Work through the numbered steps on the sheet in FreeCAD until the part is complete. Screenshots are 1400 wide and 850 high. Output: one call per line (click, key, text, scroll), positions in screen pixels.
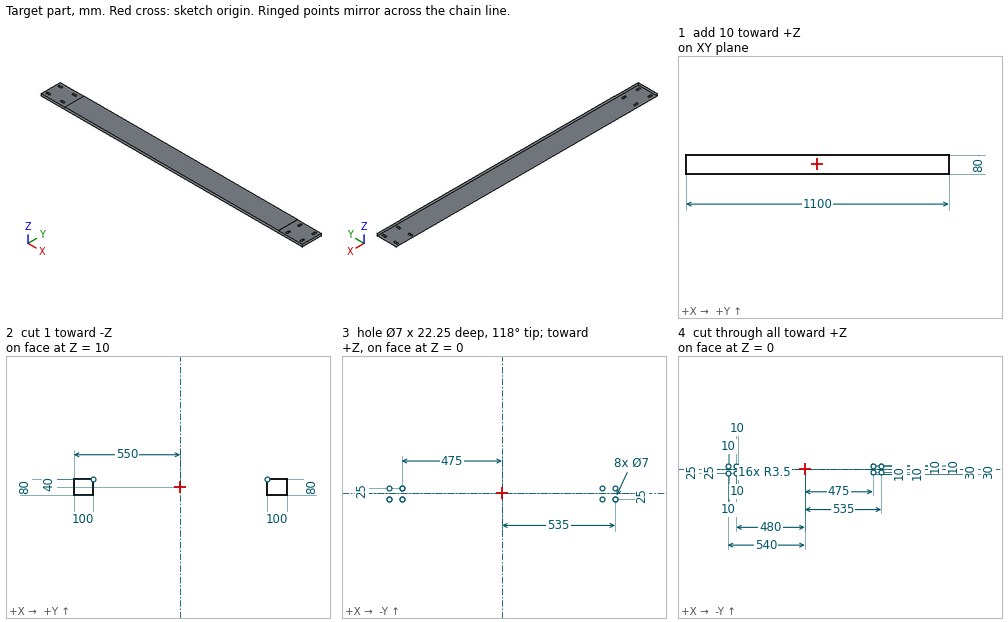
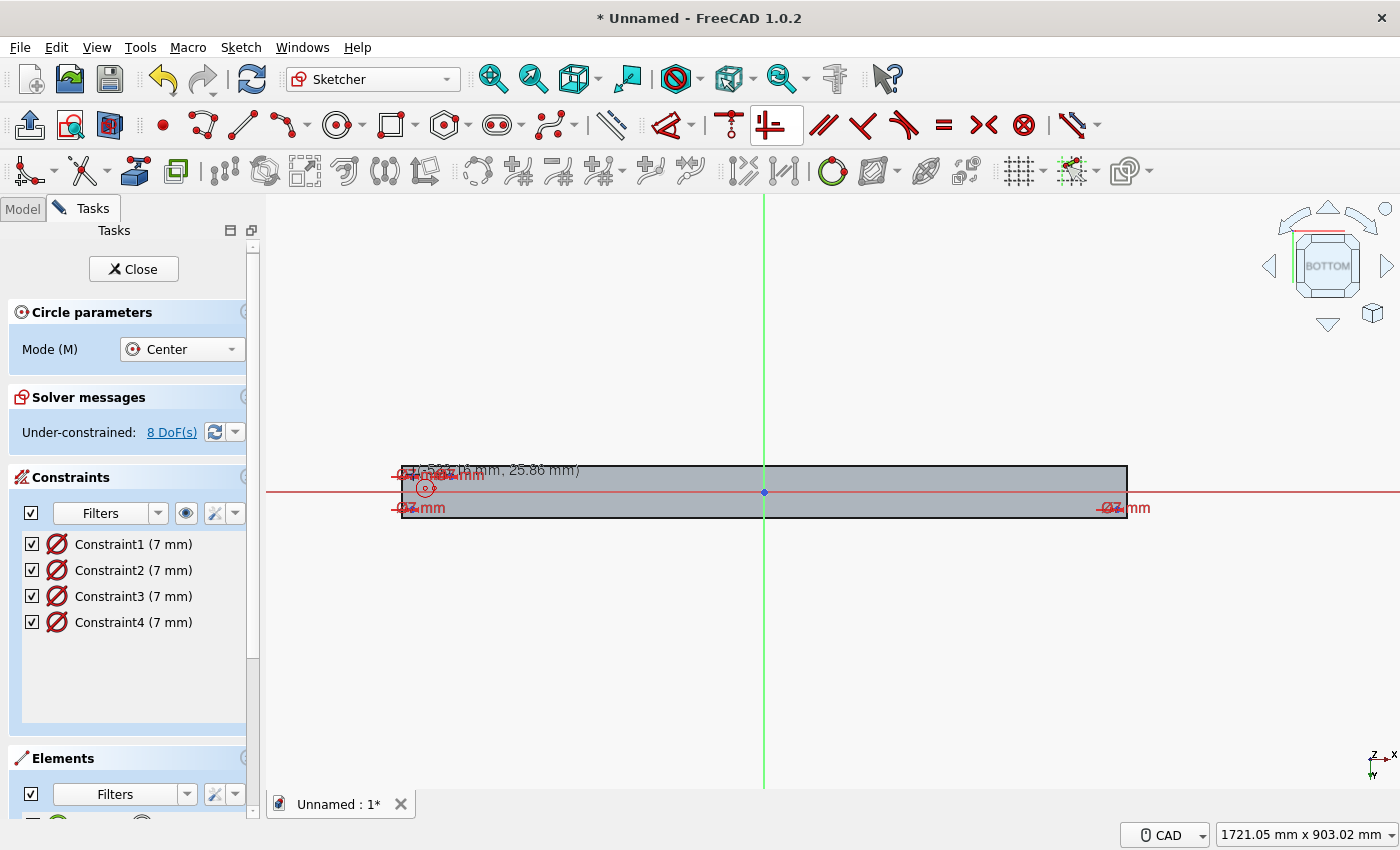
scroll(451, 509, up, 12)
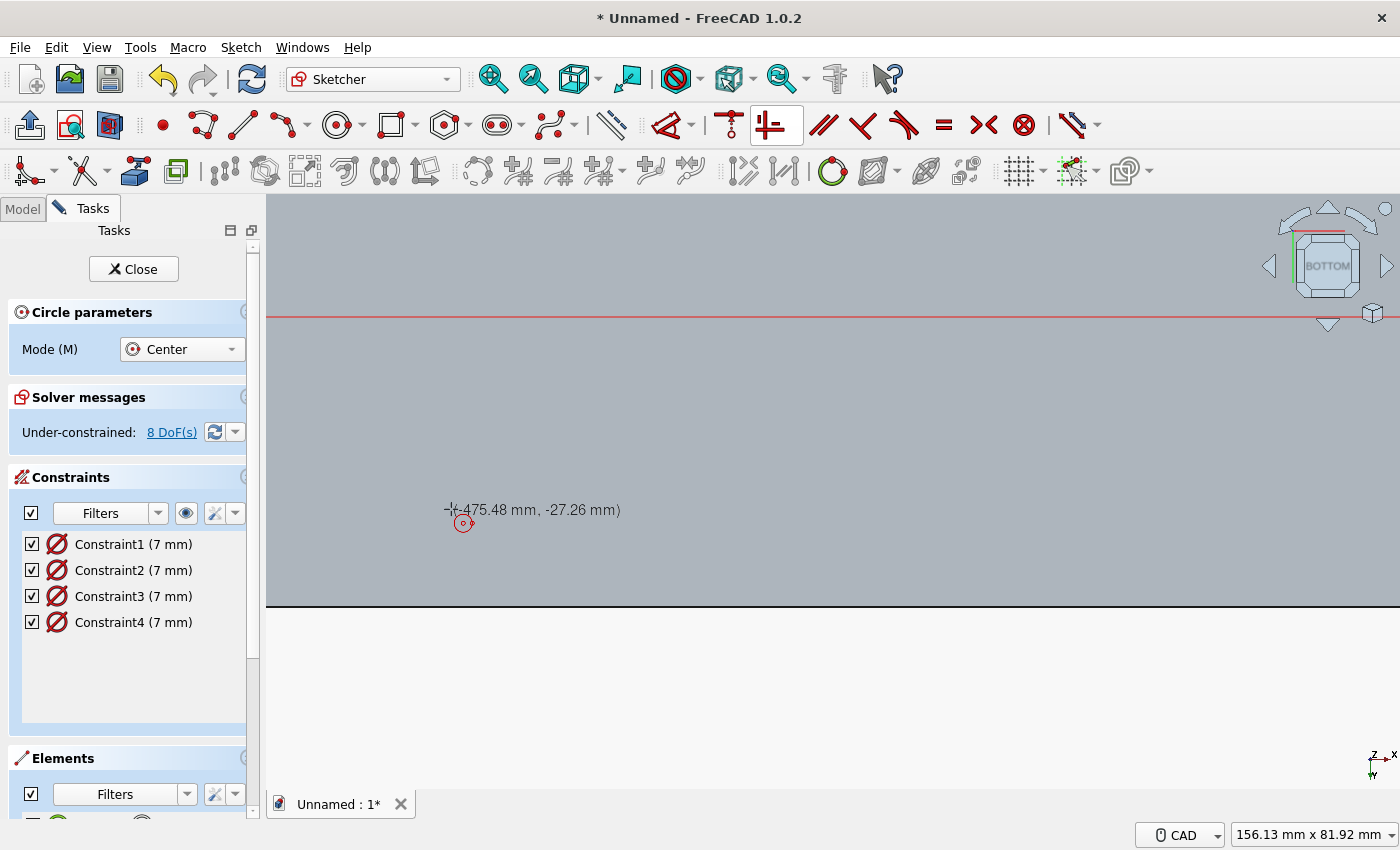
scroll(451, 509, down, 12)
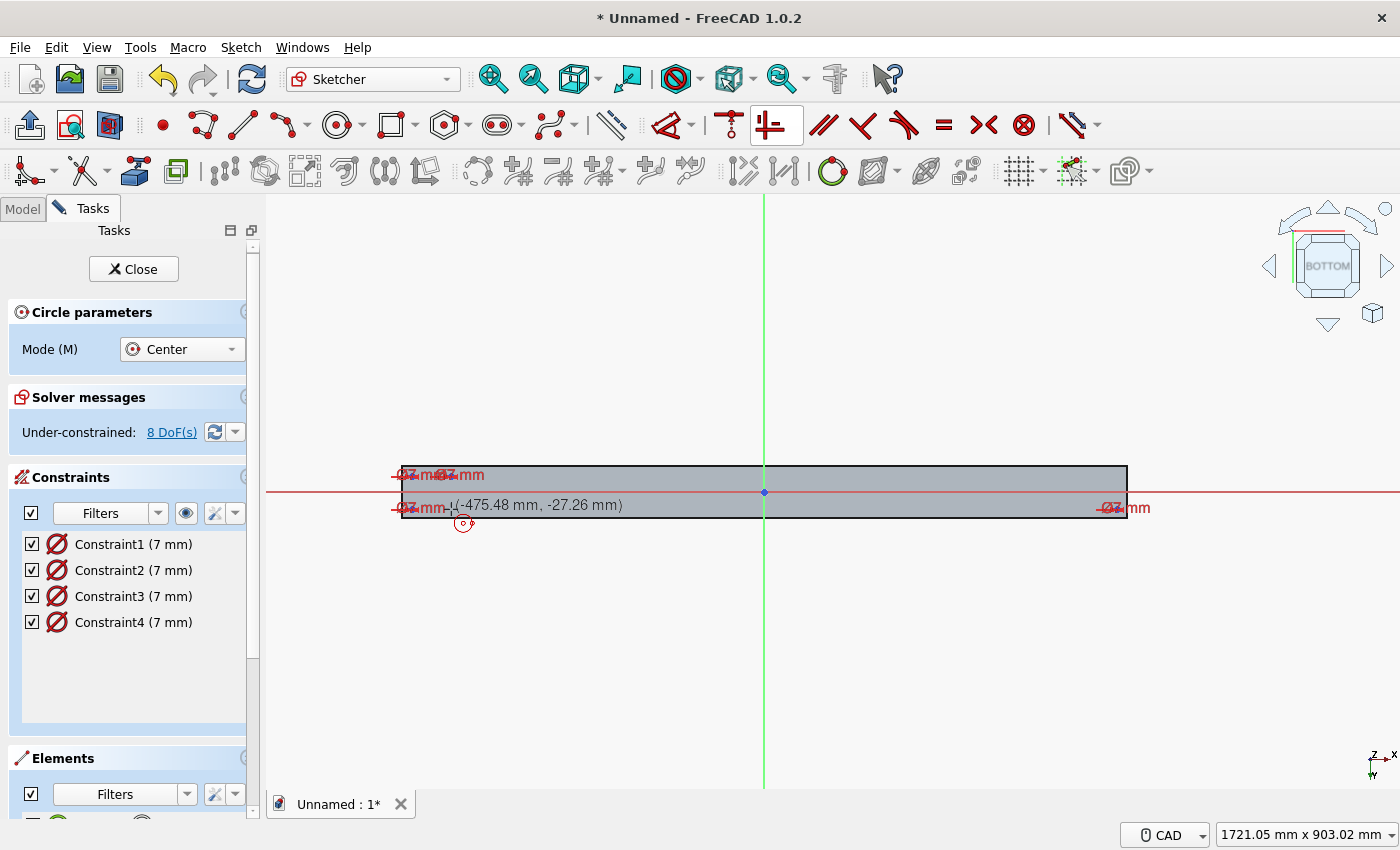
click(451, 509)
move(453, 507)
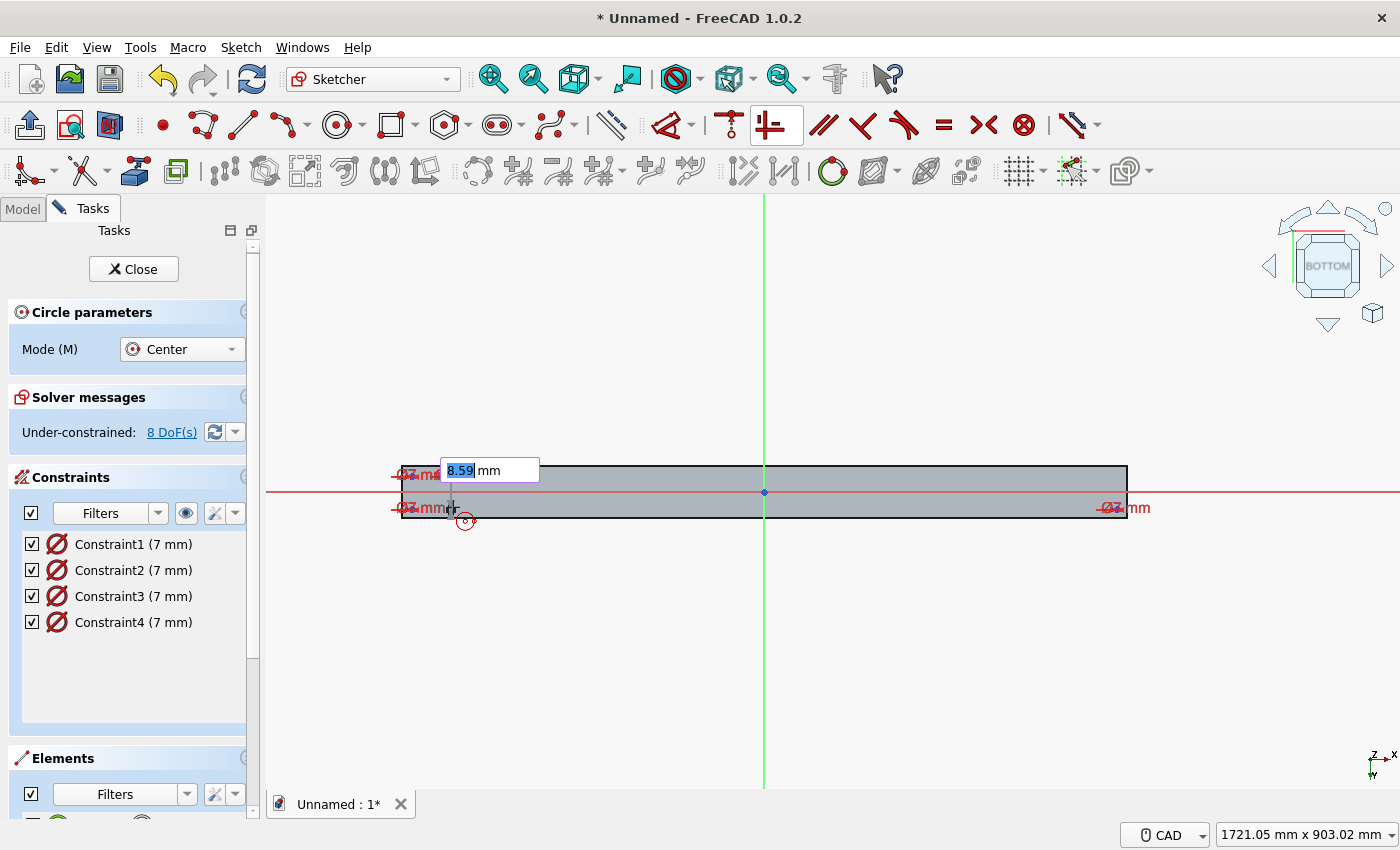
text(7)
key(Return)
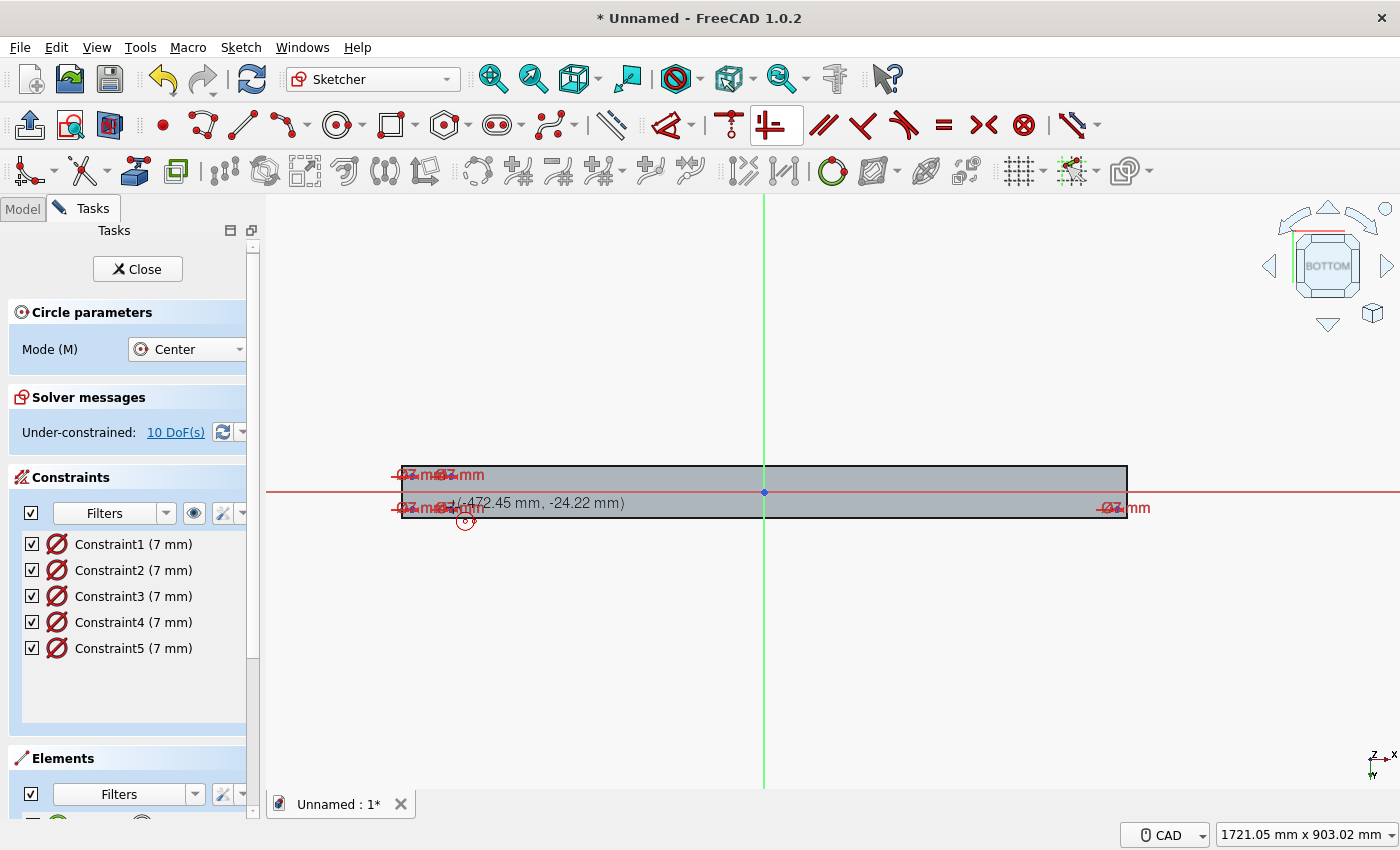
scroll(1077, 509, up, 12)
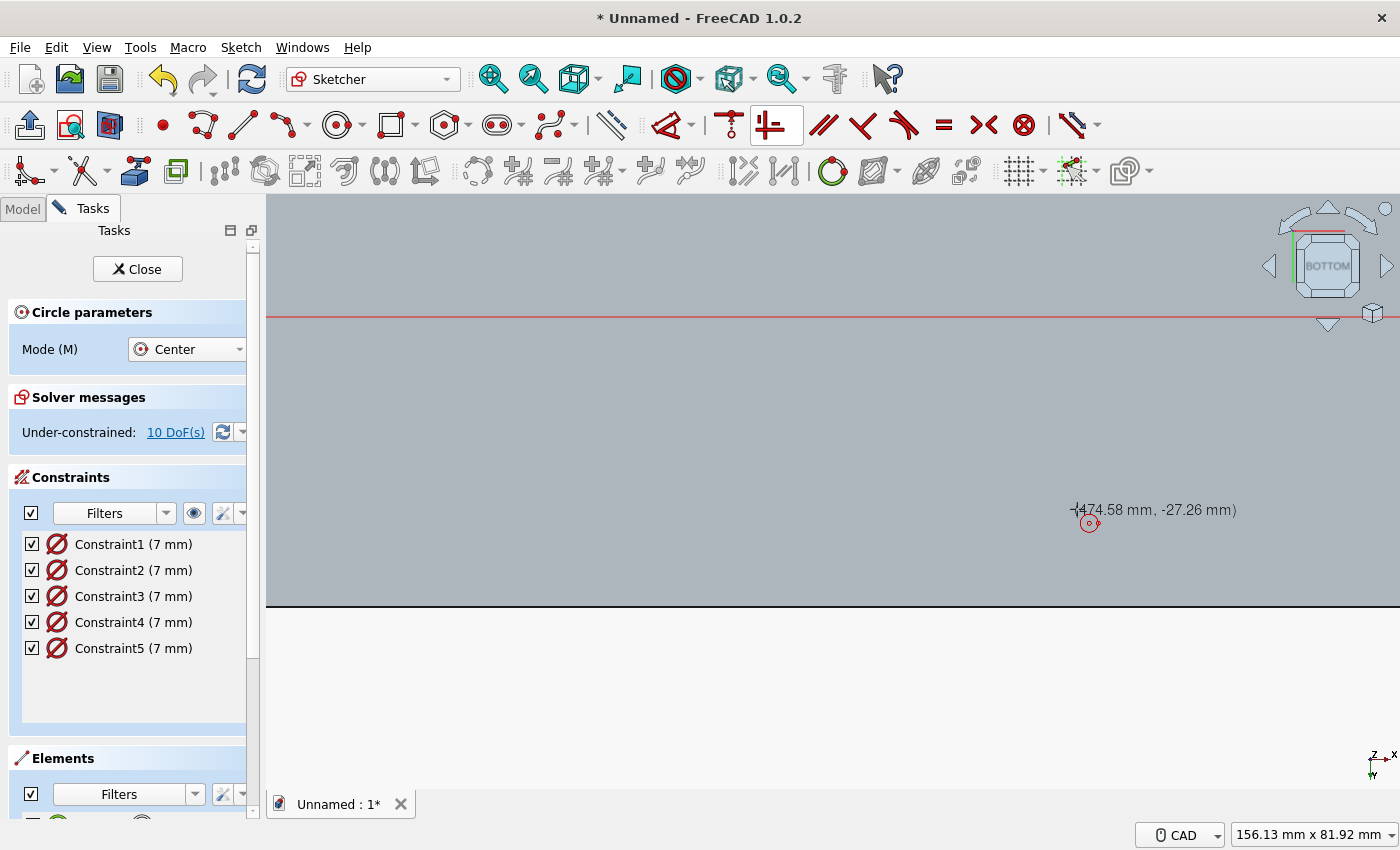
scroll(1078, 509, down, 12)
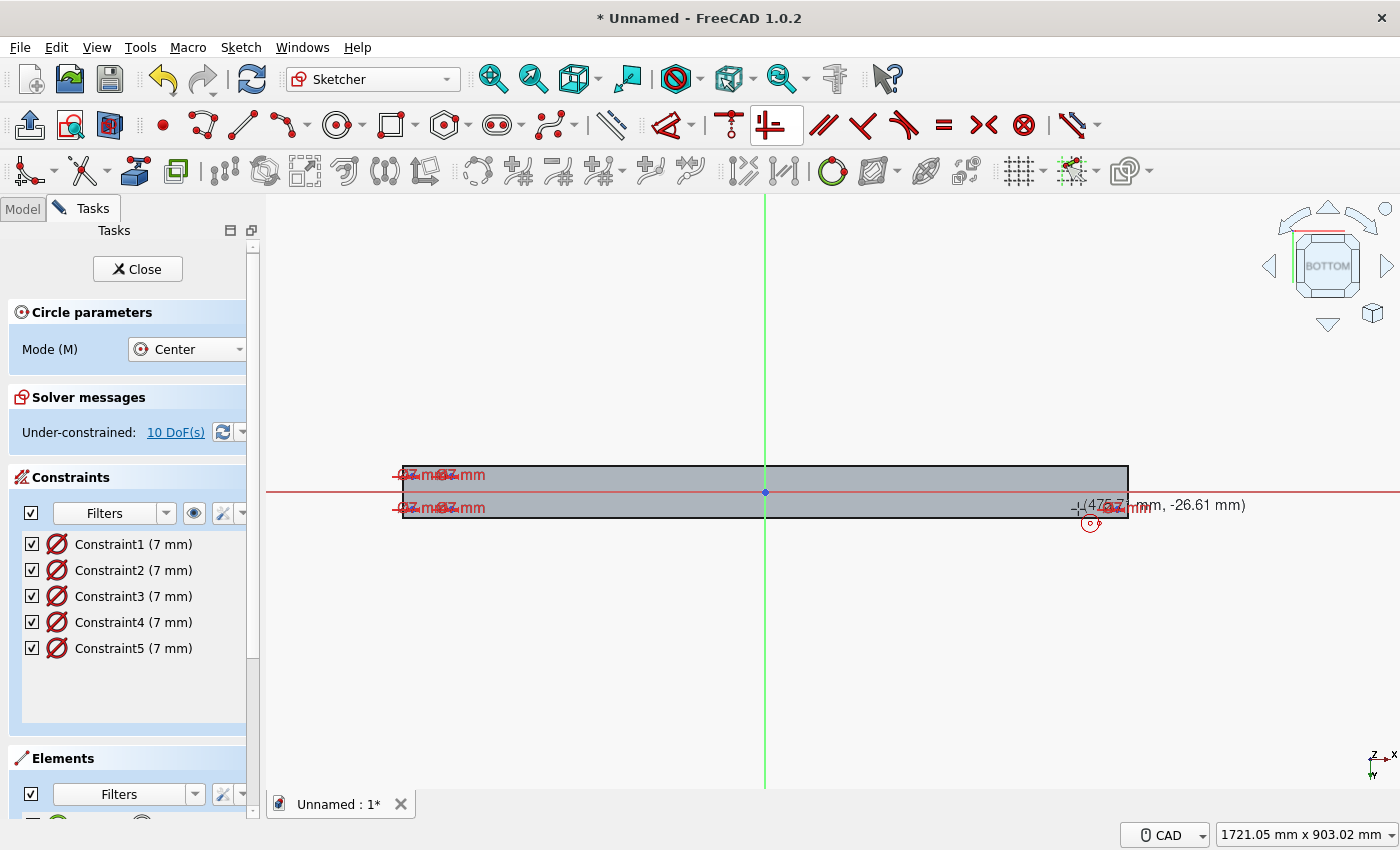
click(1078, 509)
move(1080, 507)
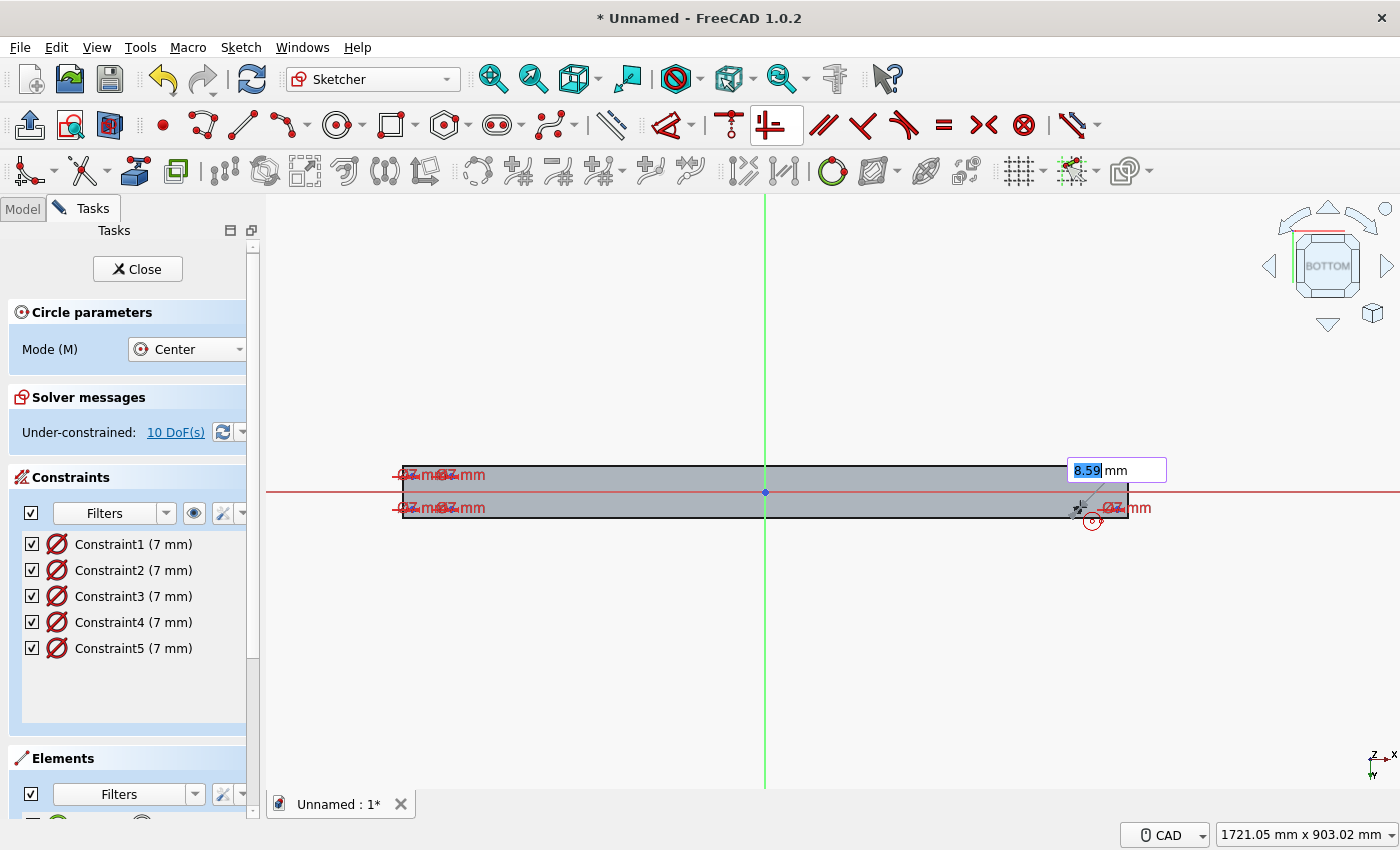
text(7)
key(Return)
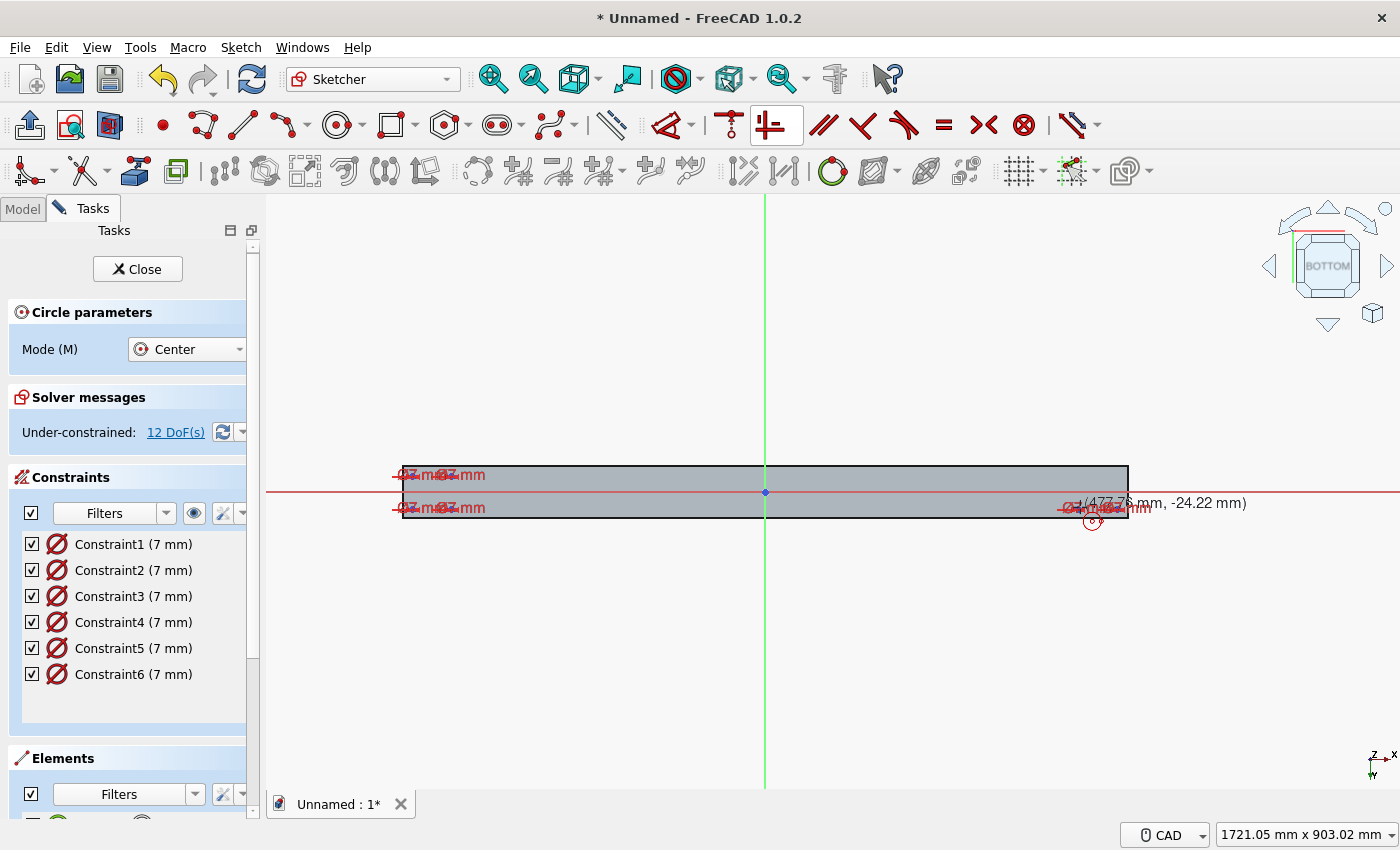
scroll(1078, 476, up, 12)